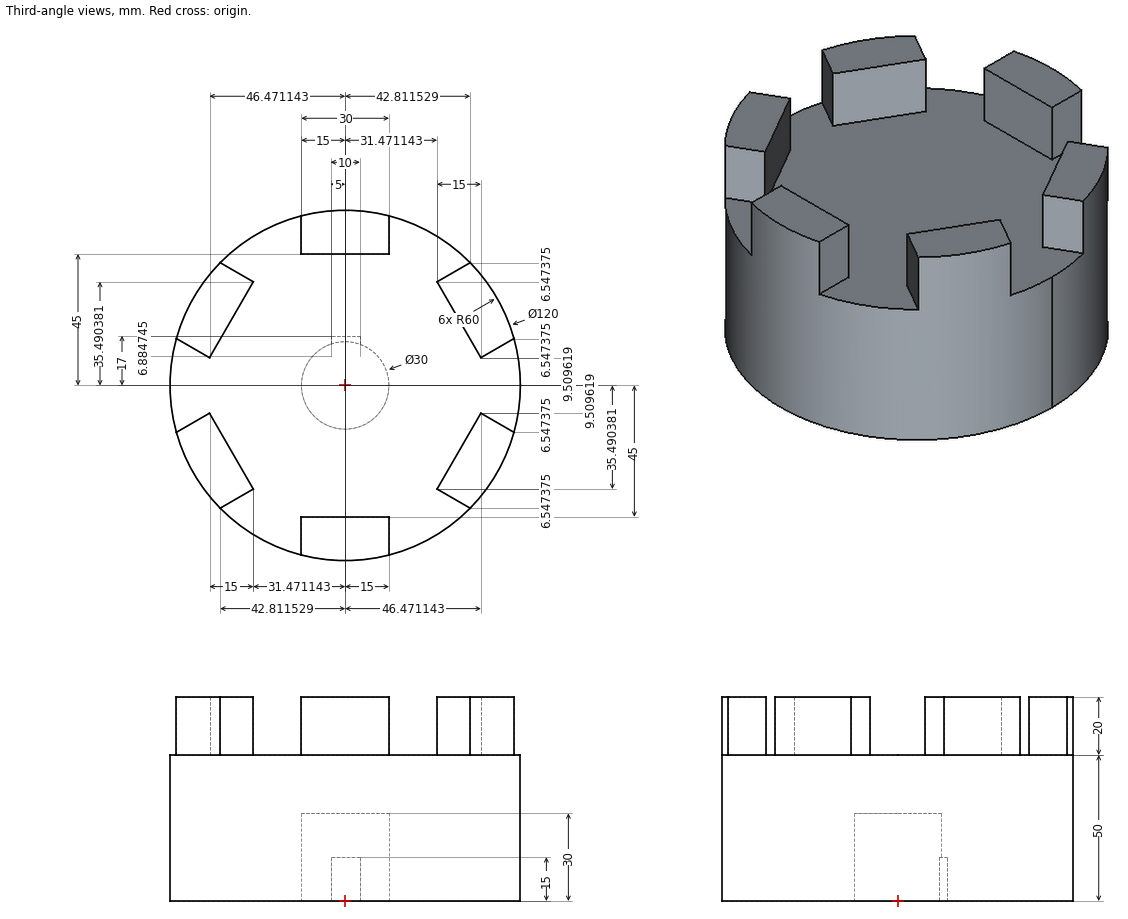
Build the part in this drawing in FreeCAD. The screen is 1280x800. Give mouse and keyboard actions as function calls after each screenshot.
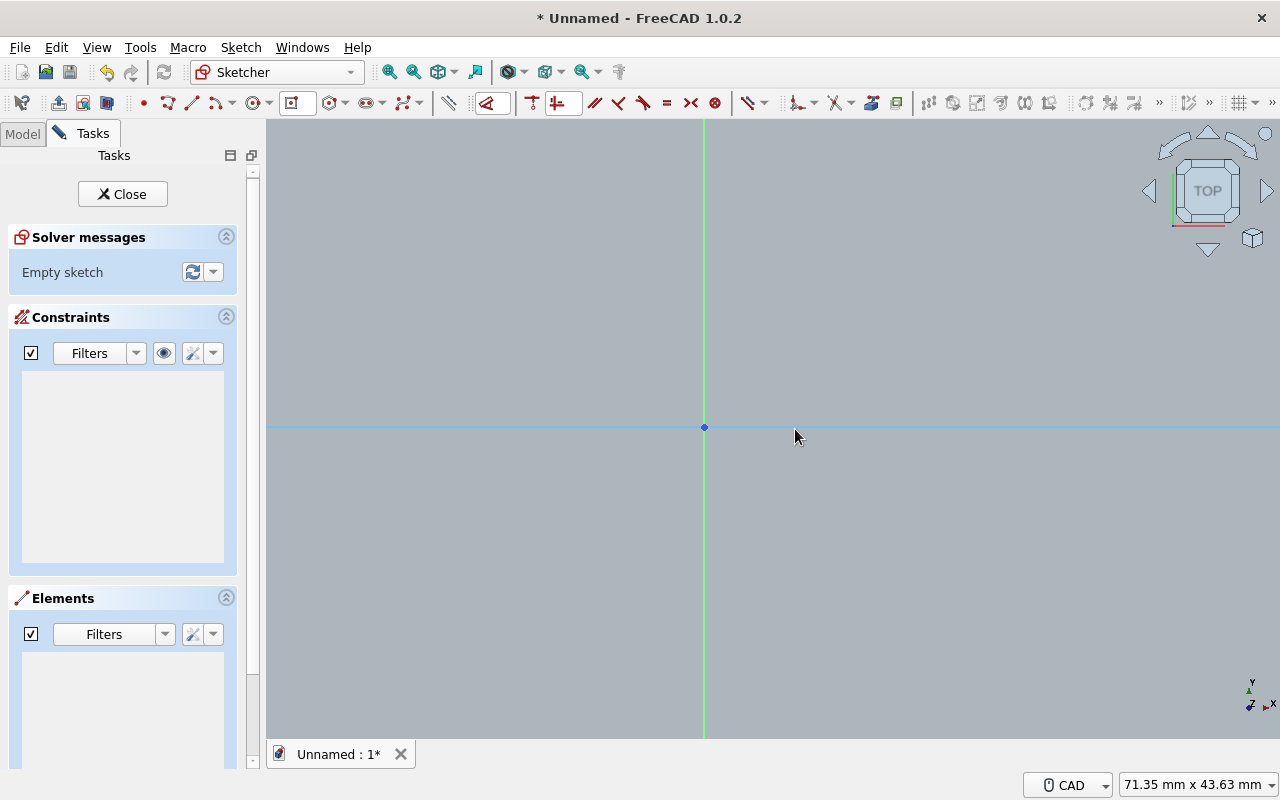
key(g)
key(c)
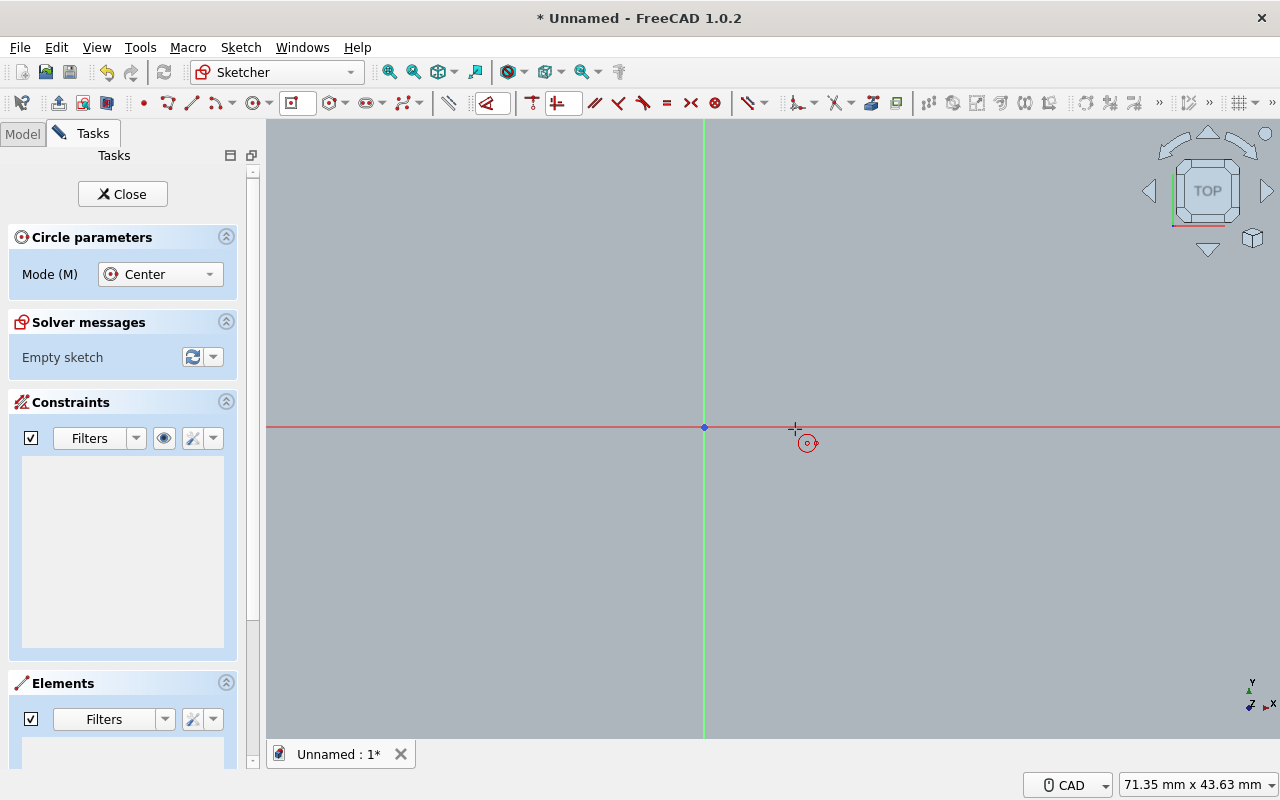
click(704, 427)
click(855, 277)
key(Escape)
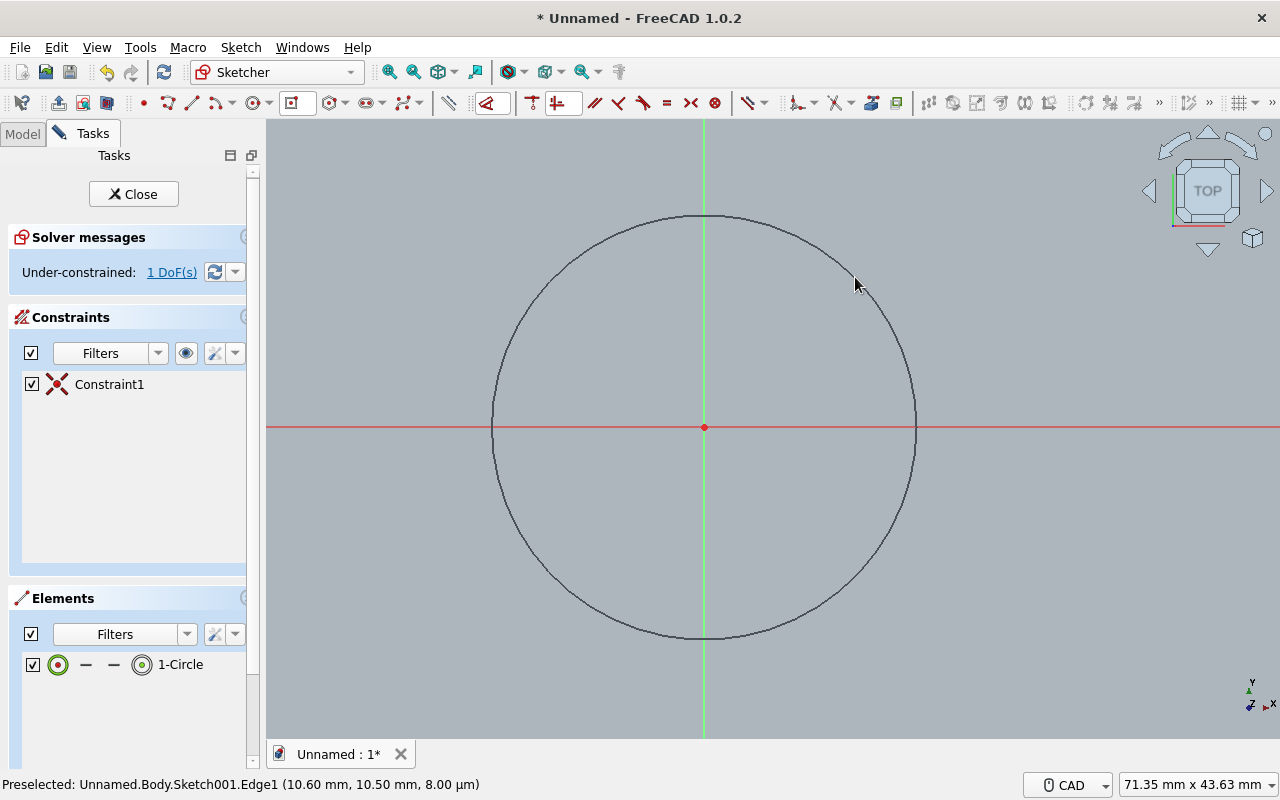
click(854, 277)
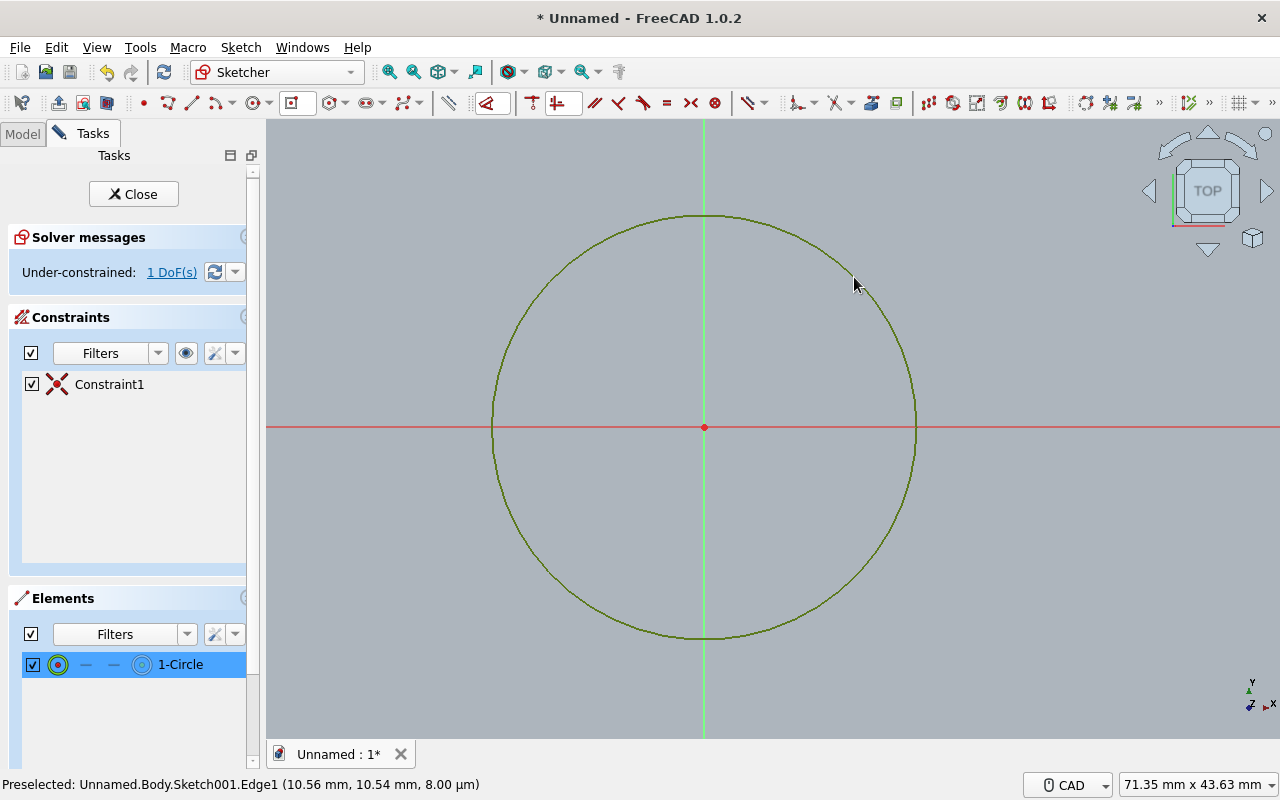
key(k)
key(o)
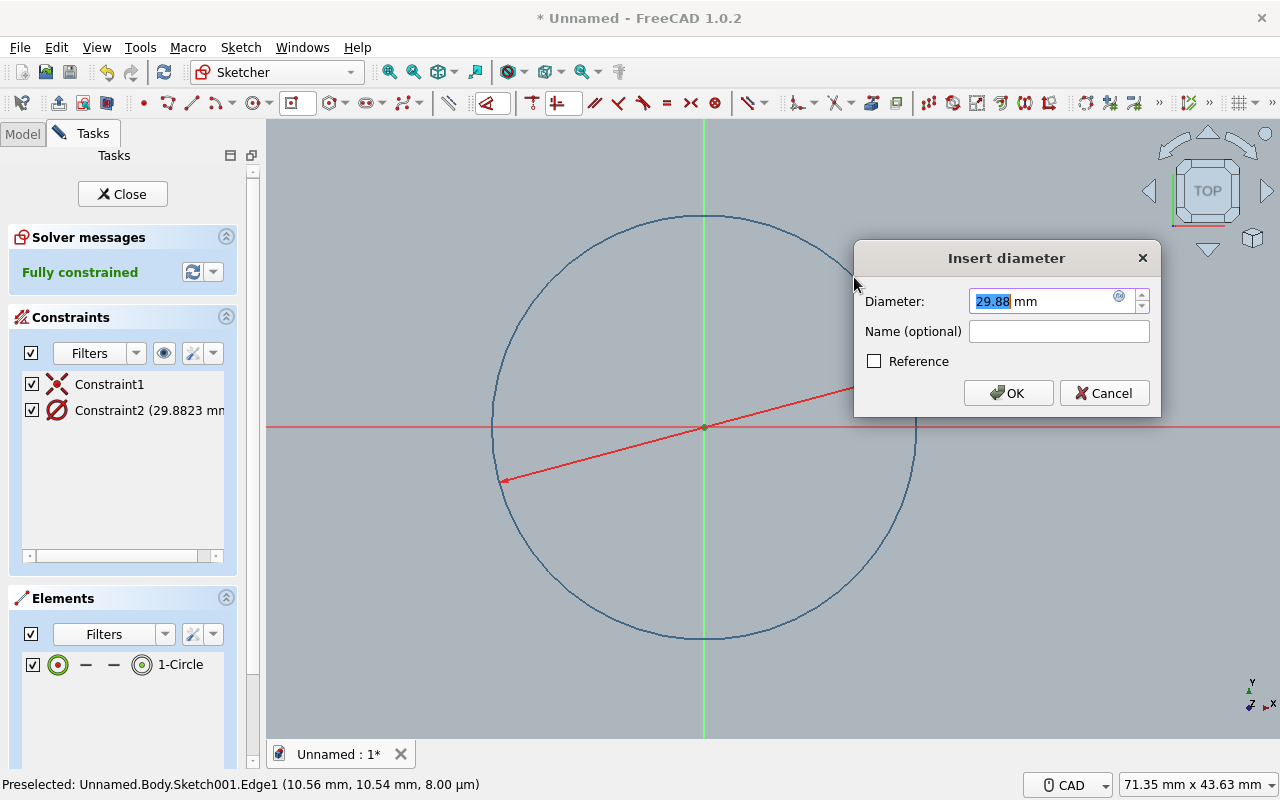
text(30)
key(Return)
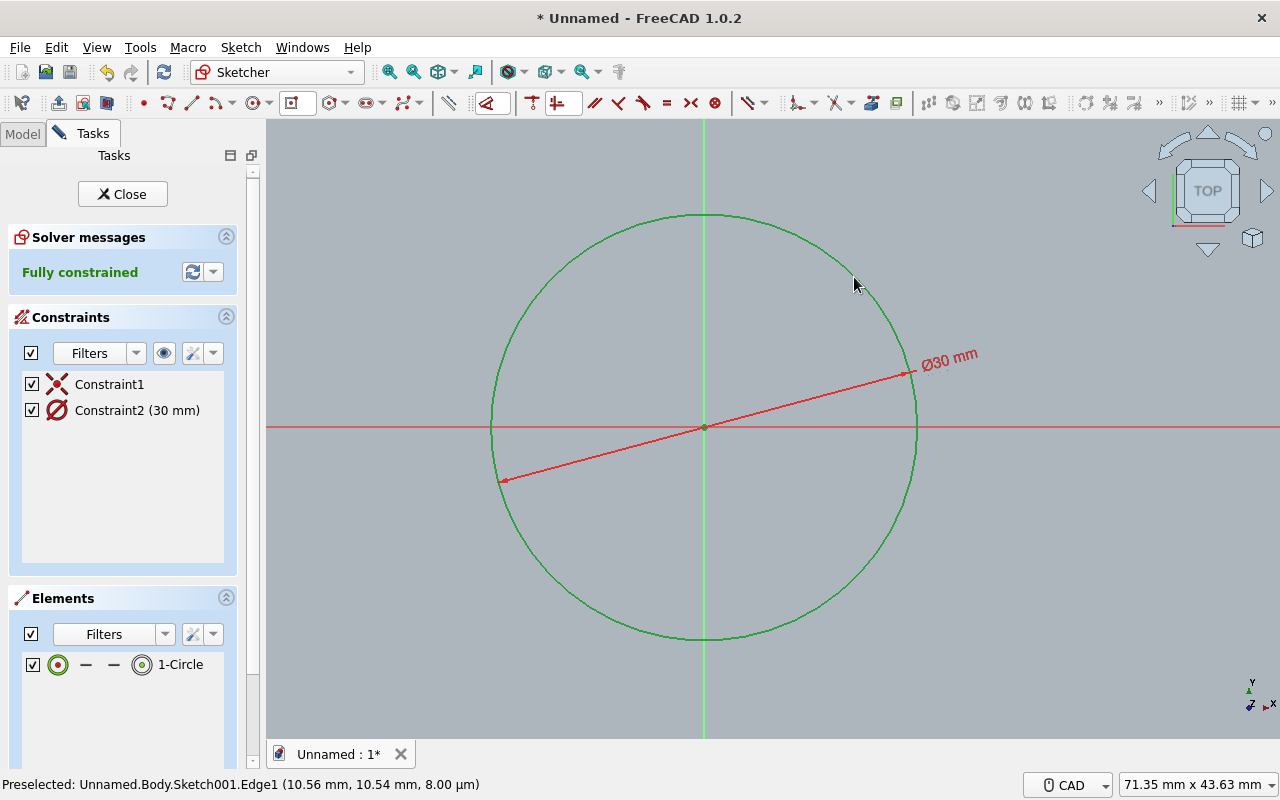
click(123, 194)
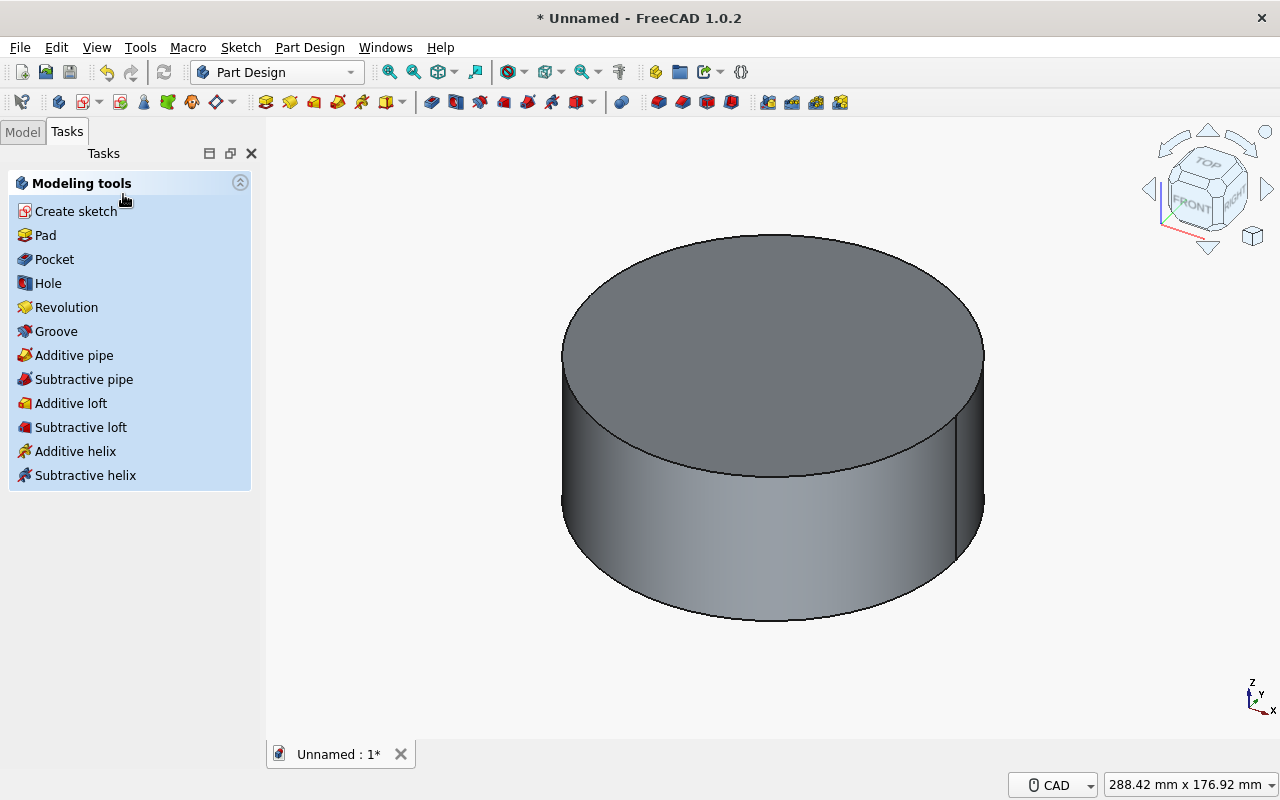
click(432, 102)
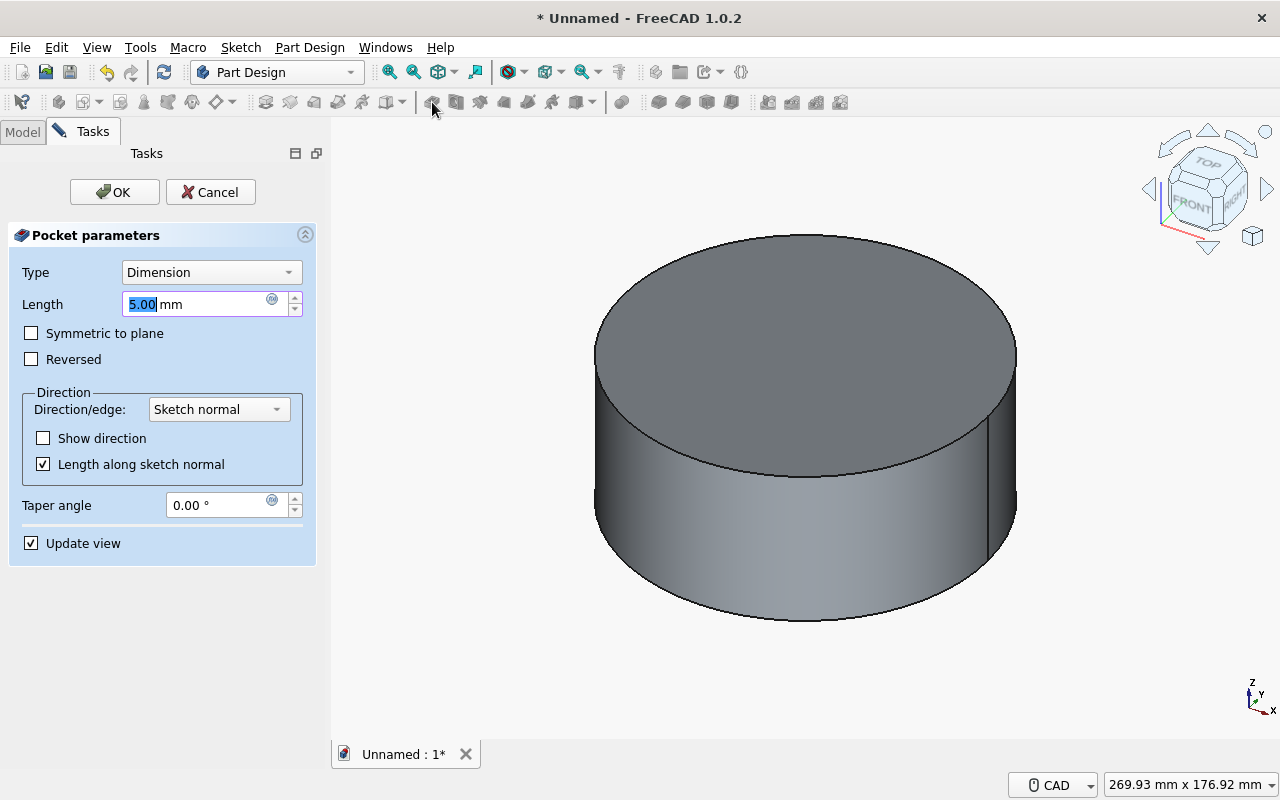
text(30)
key(Tab)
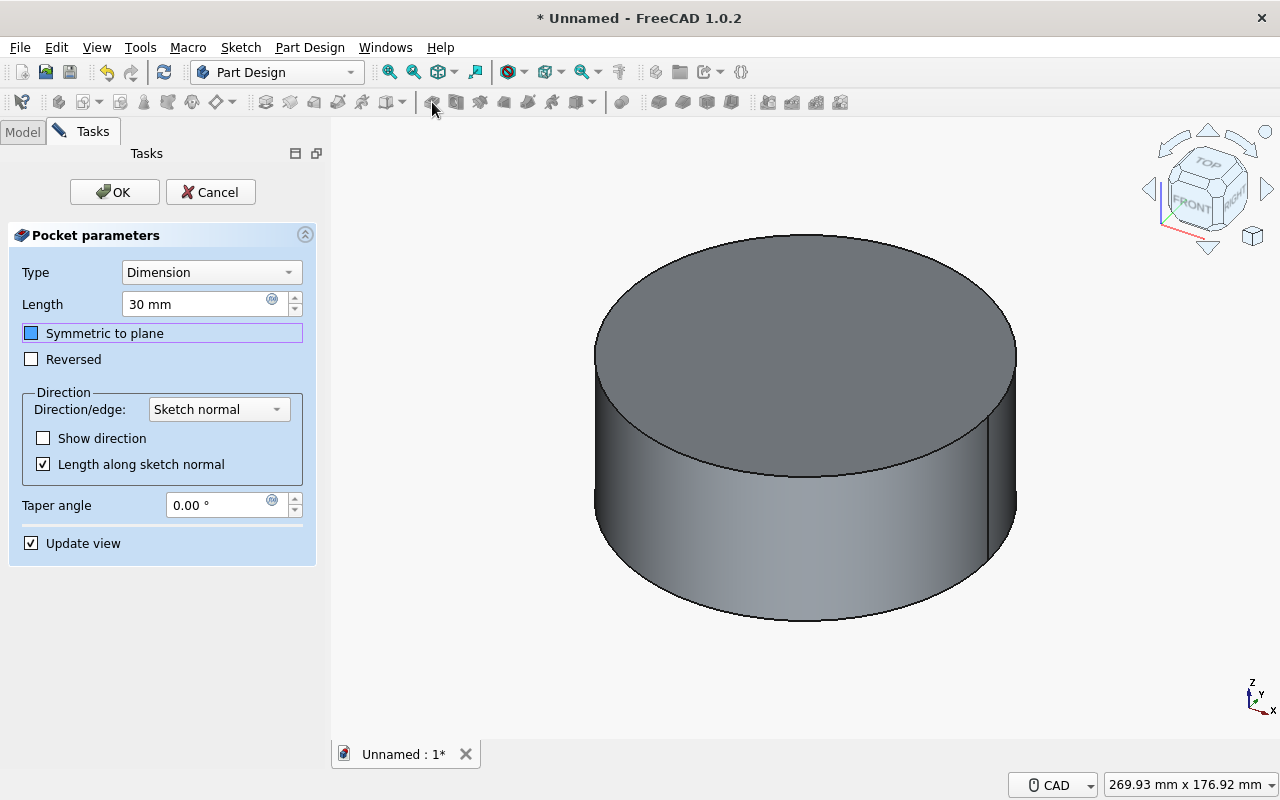
click(30, 359)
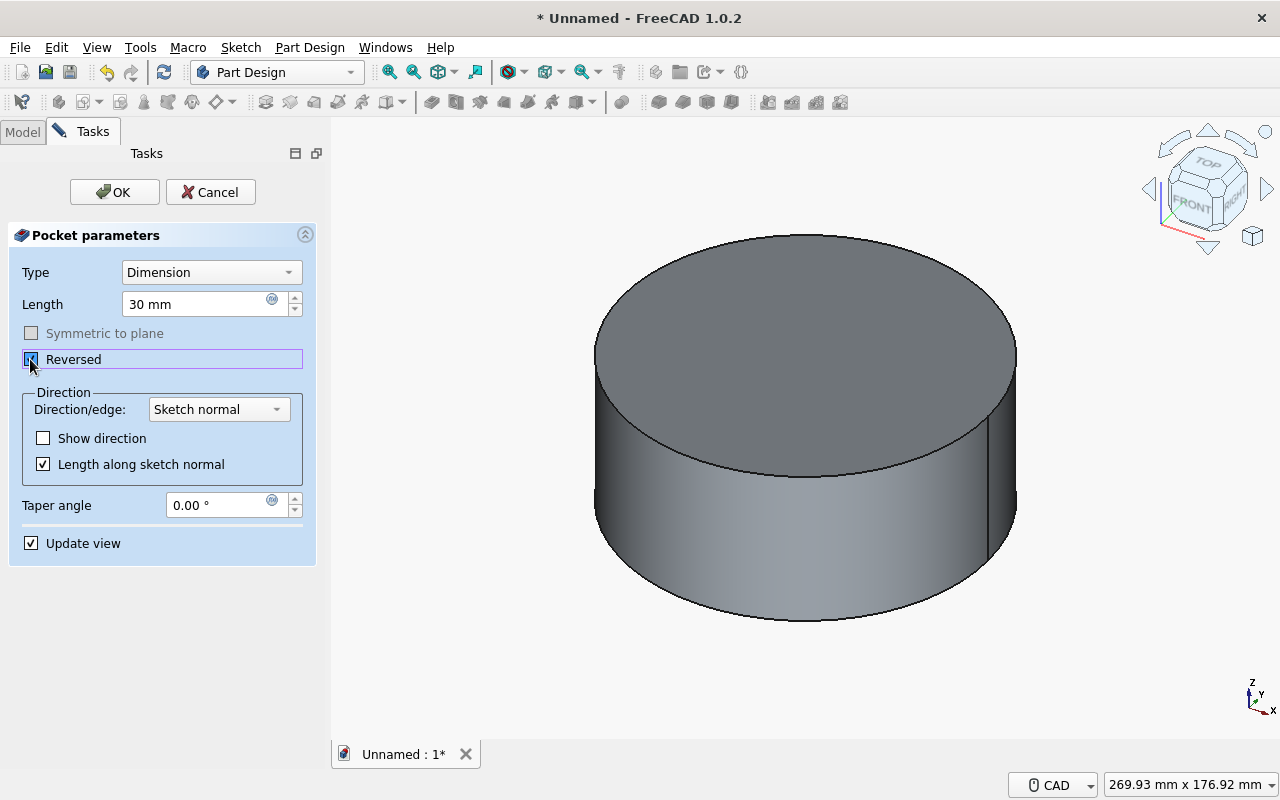
click(115, 192)